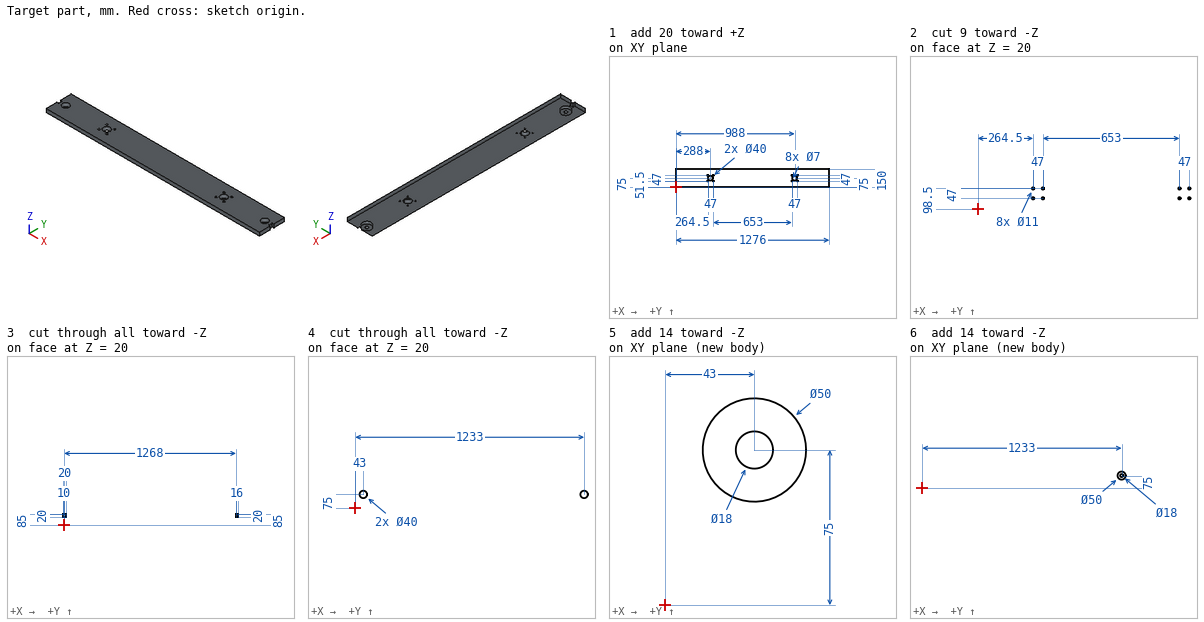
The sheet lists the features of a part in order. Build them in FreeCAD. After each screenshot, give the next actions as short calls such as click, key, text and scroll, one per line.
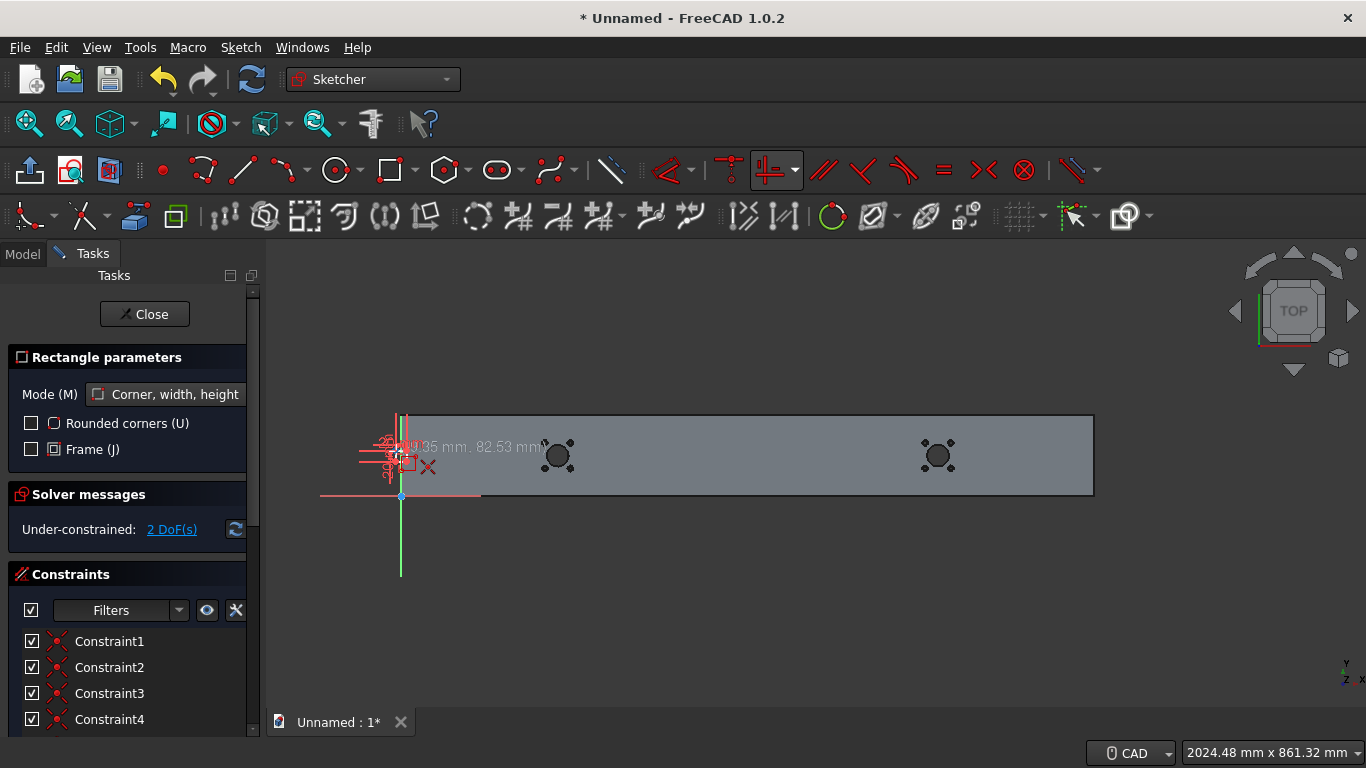
scroll(1090, 450, up, 4)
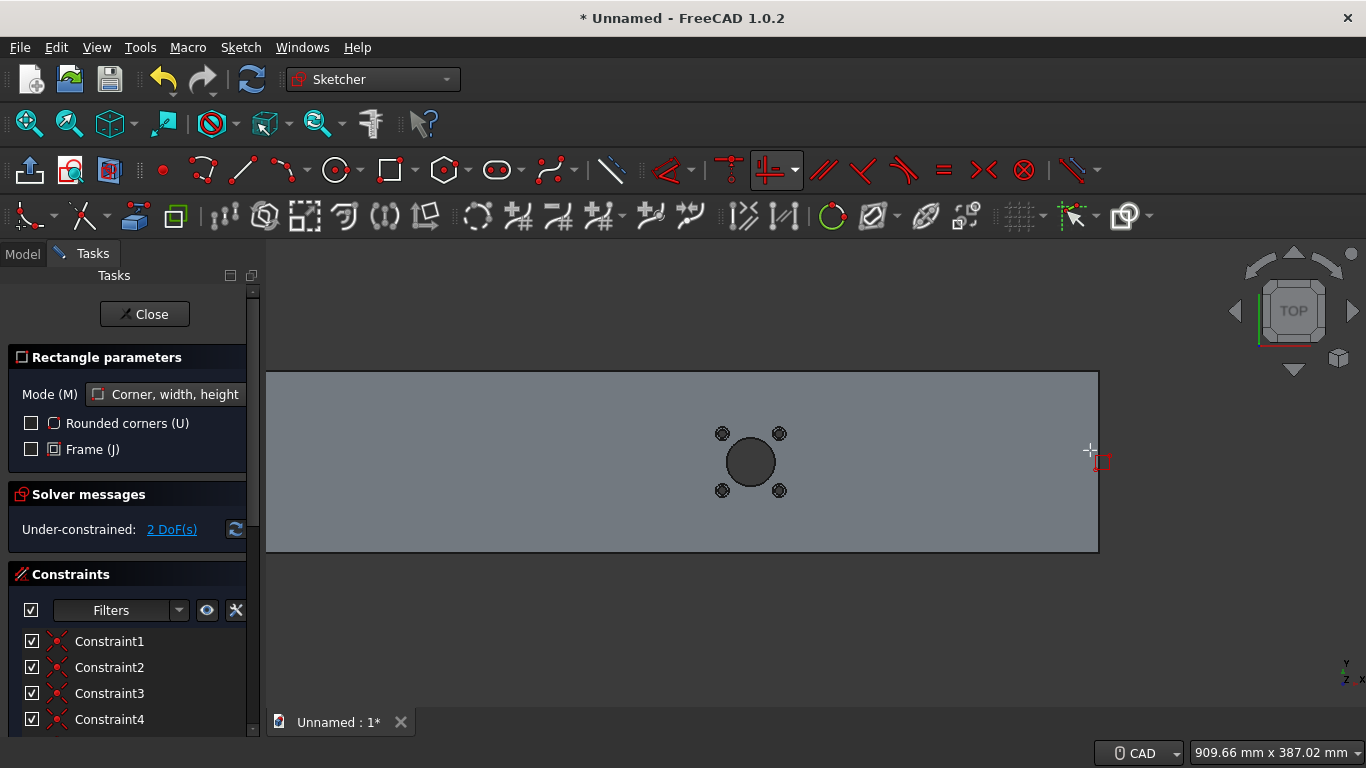
click(1089, 450)
move(1109, 474)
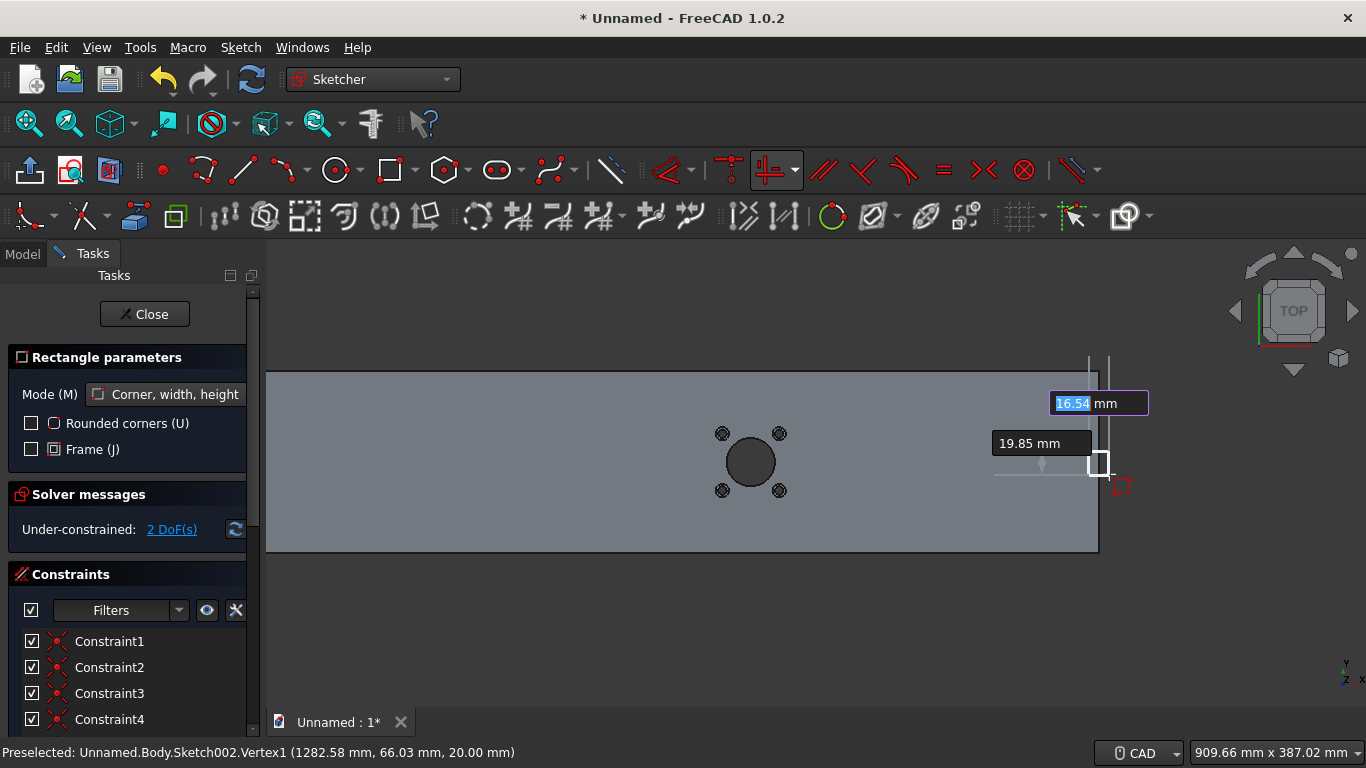
text(16)
key(Tab)
text(20)
key(Return)
key(Escape)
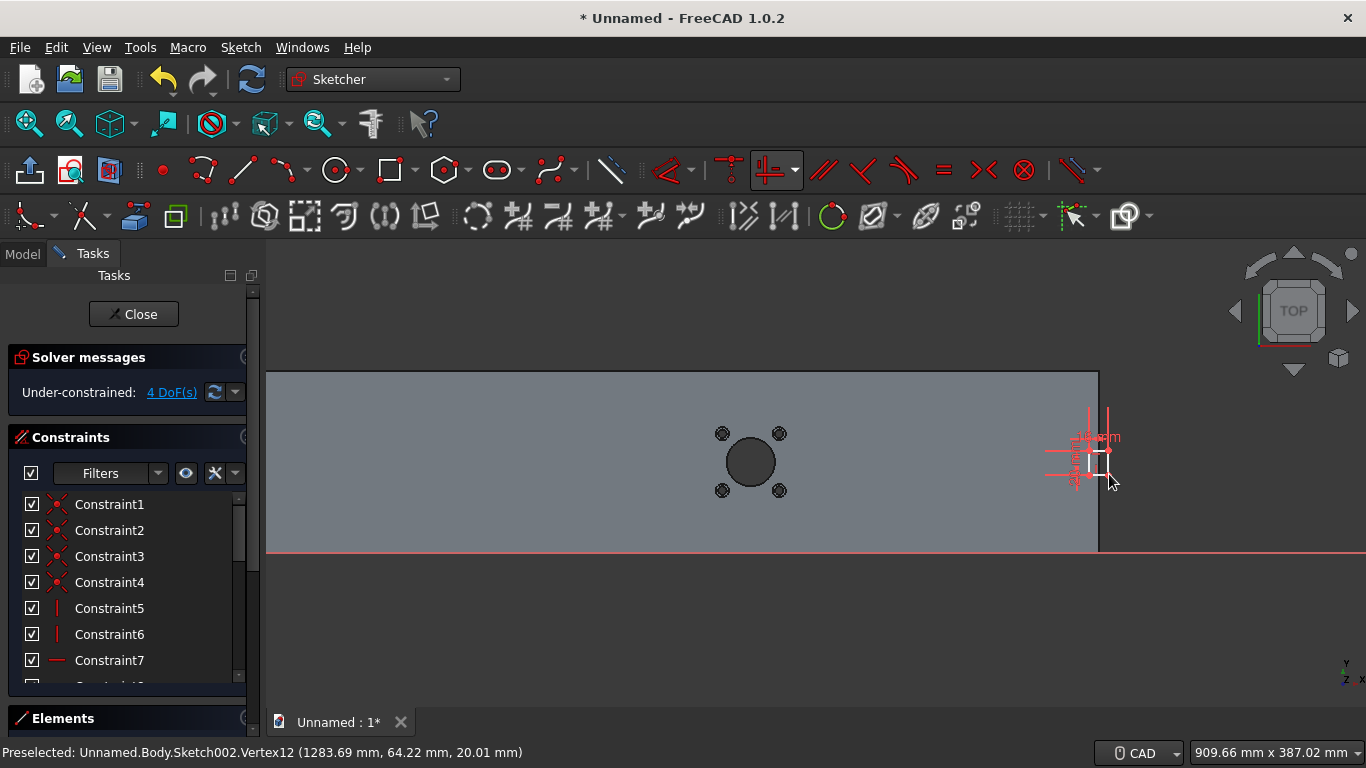
click(666, 170)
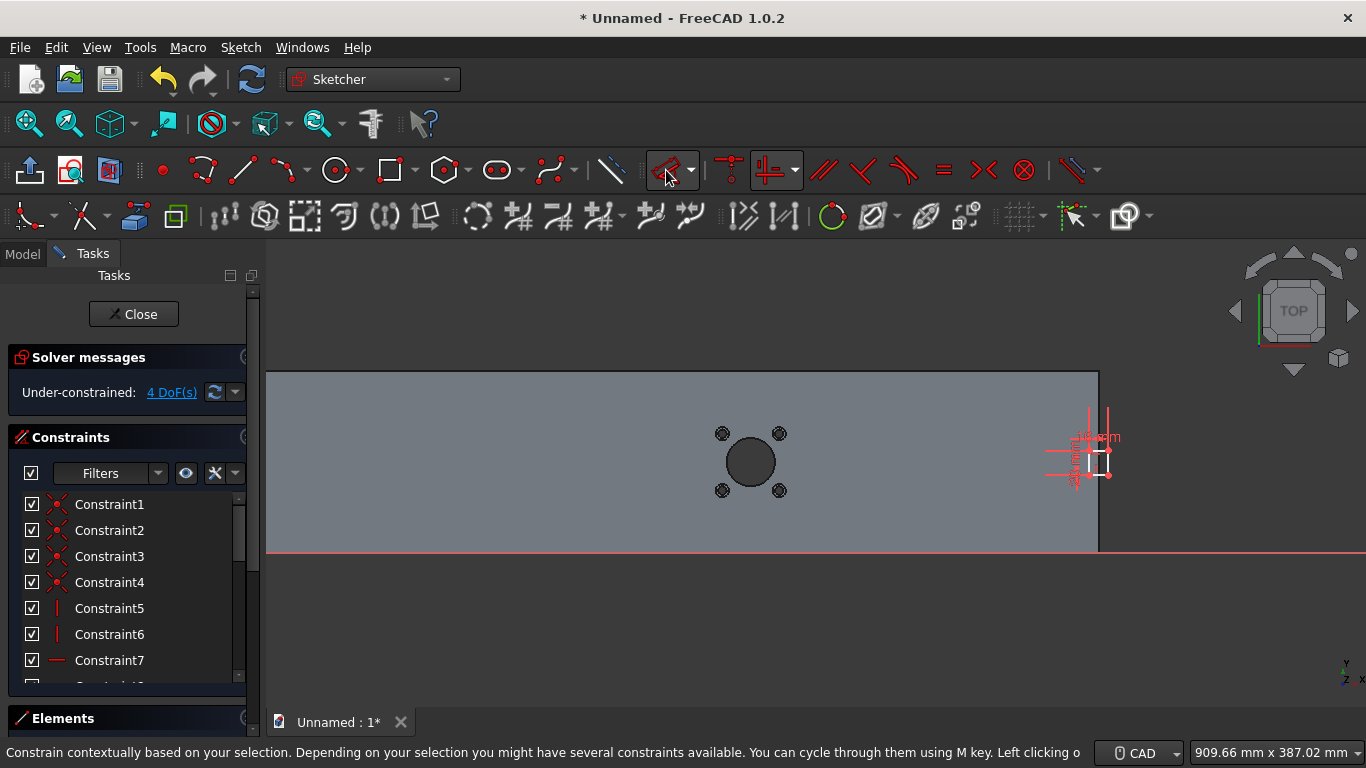
scroll(1091, 450, down, 4)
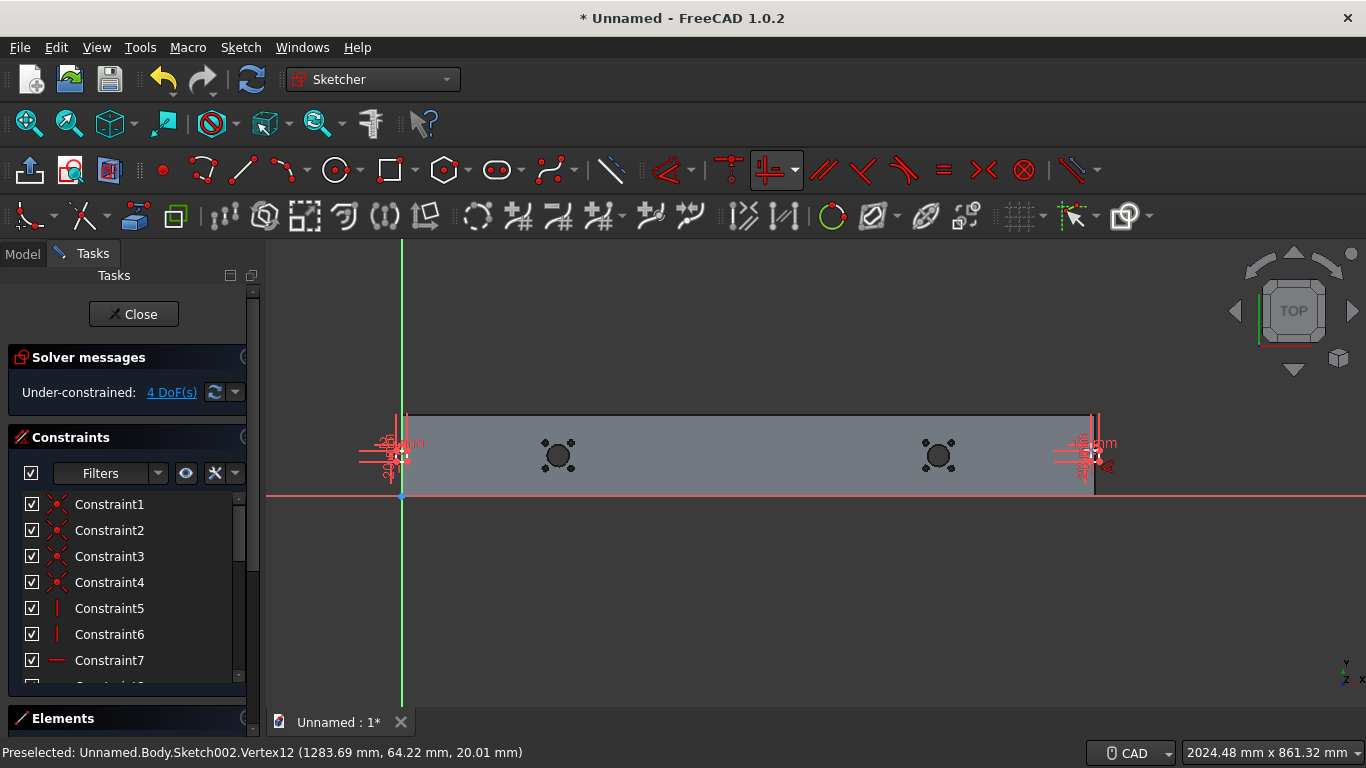
scroll(396, 451, up, 10)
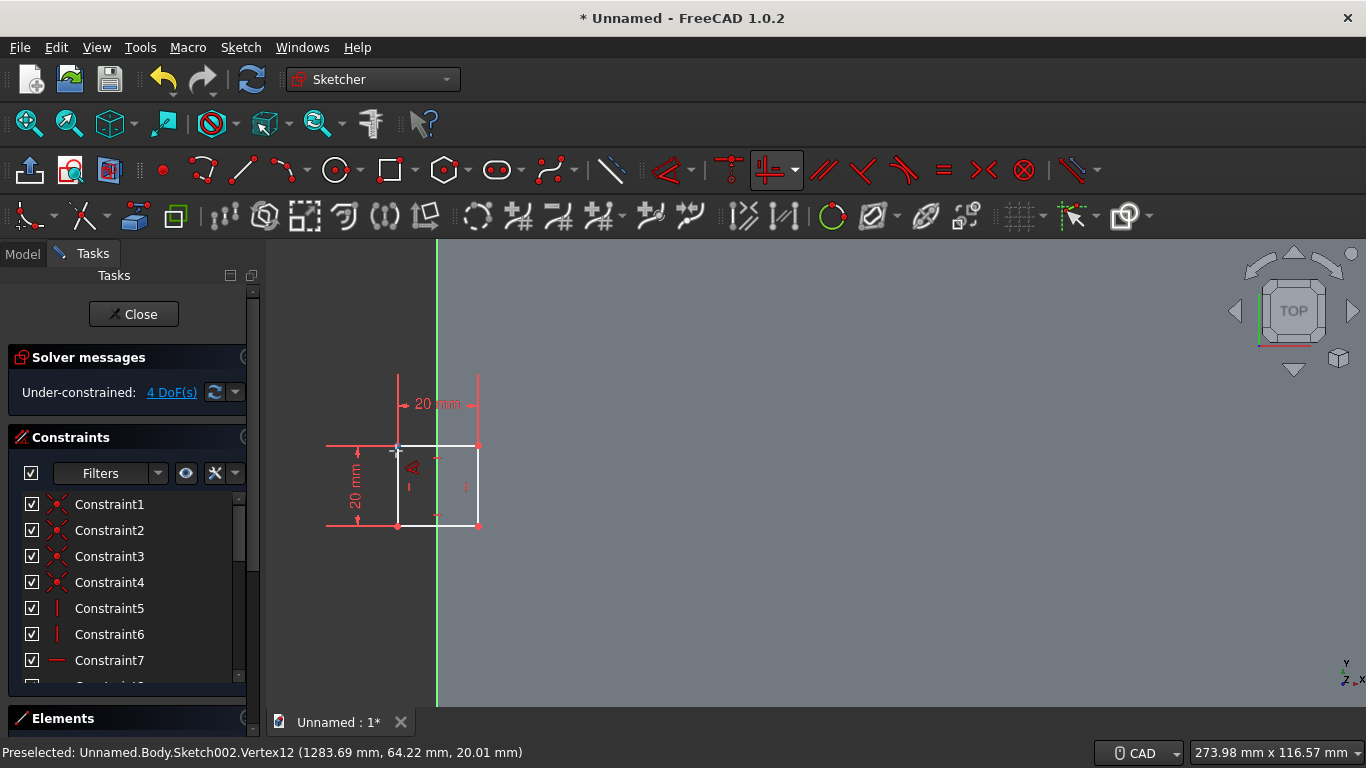
click(398, 446)
click(418, 412)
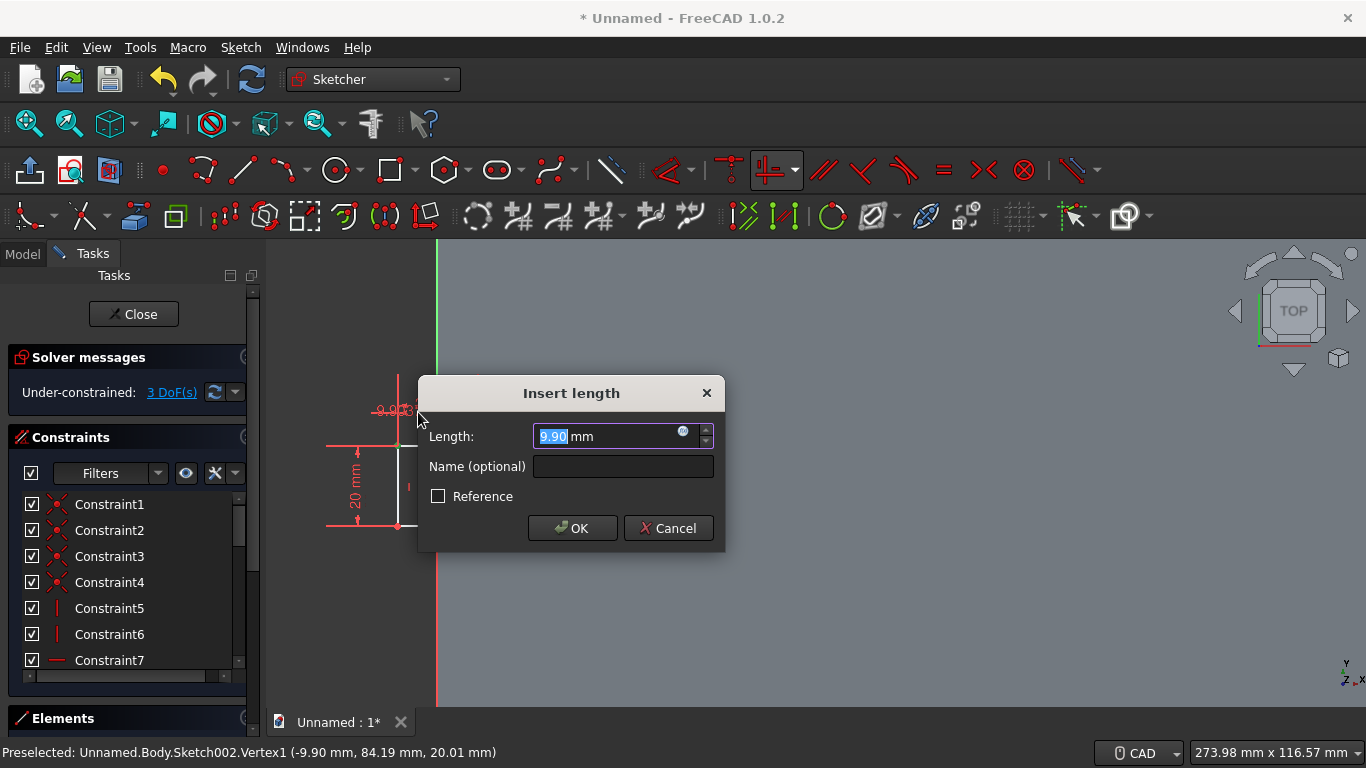
text(10)
key(Return)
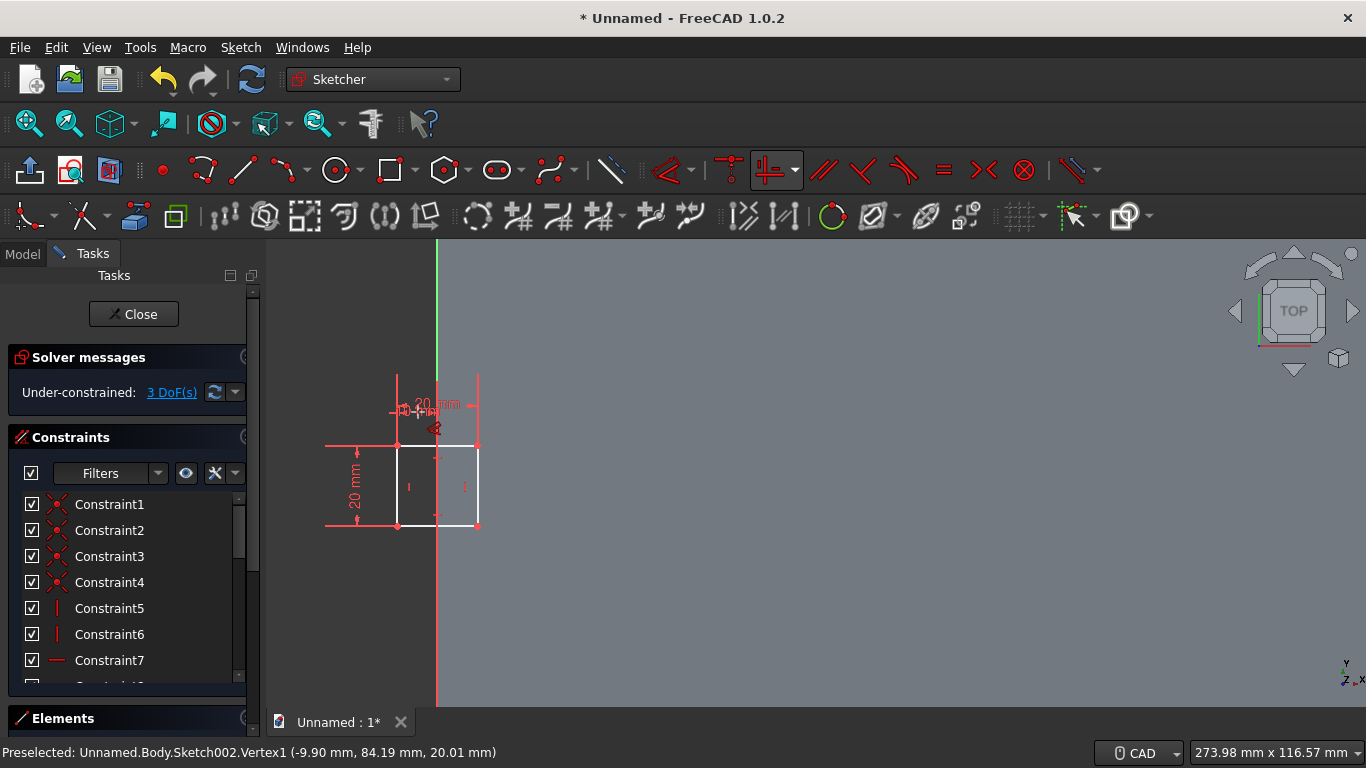
scroll(396, 451, down, 10)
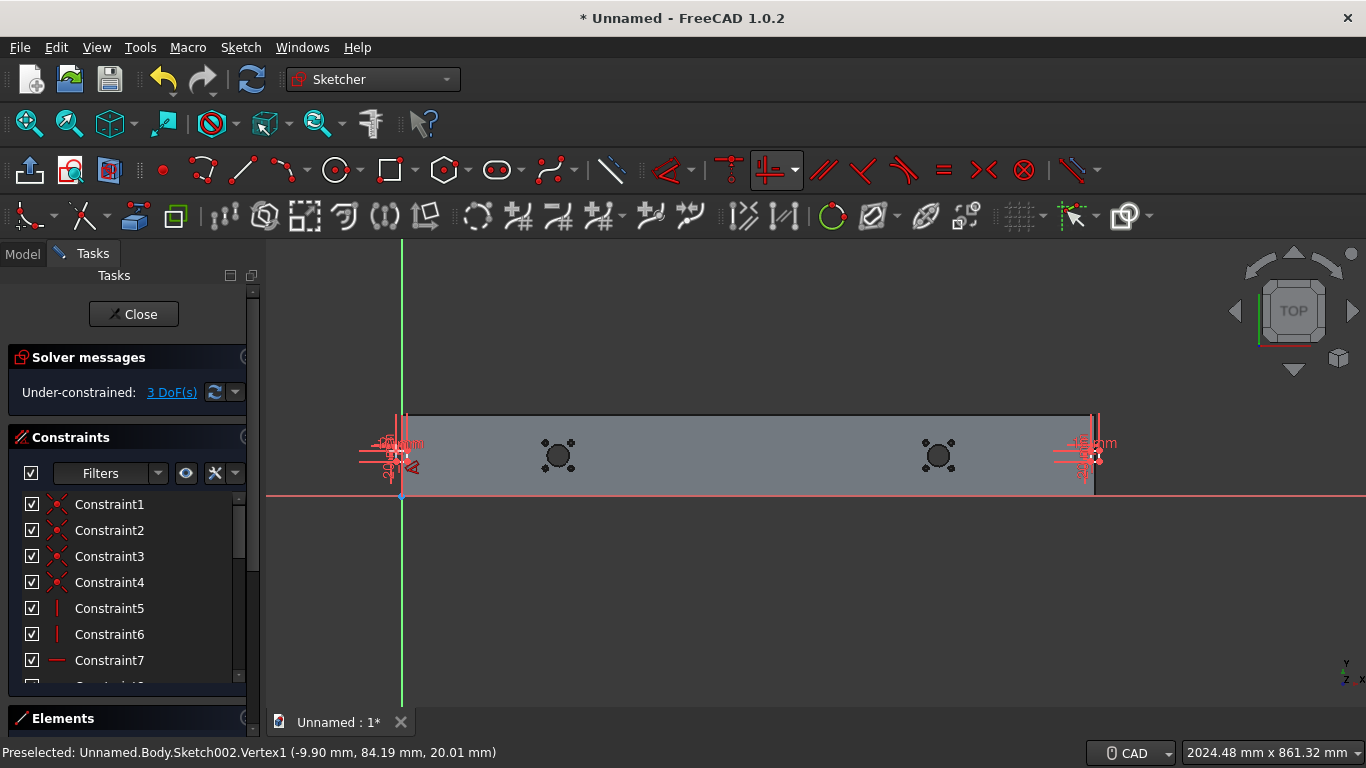
click(396, 451)
click(362, 474)